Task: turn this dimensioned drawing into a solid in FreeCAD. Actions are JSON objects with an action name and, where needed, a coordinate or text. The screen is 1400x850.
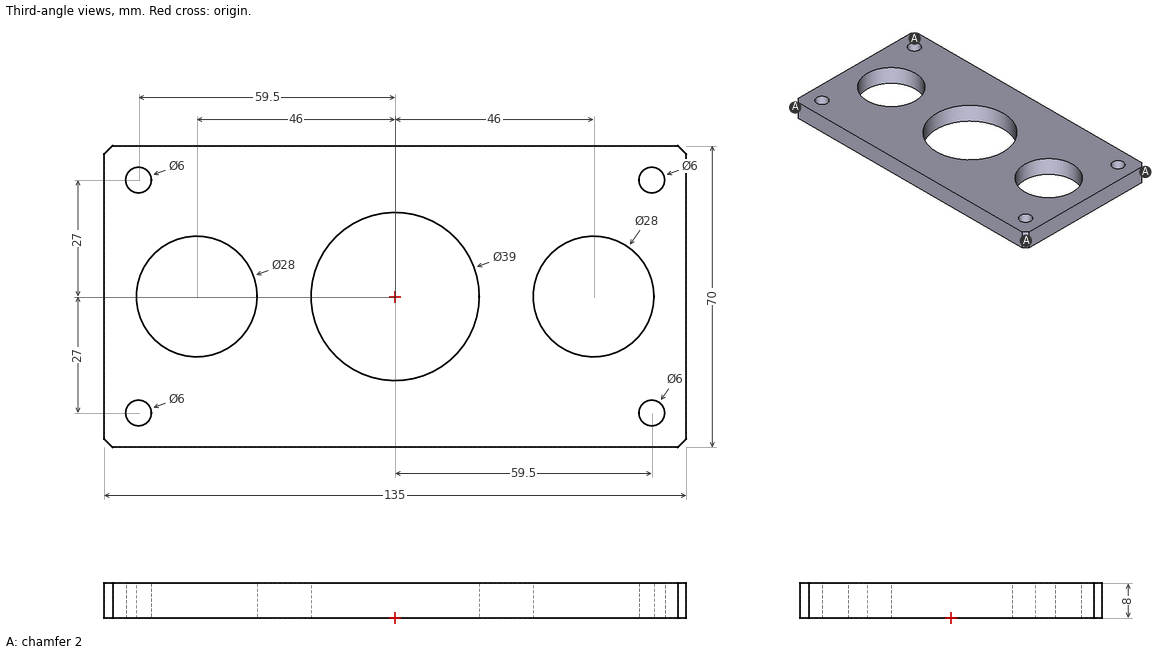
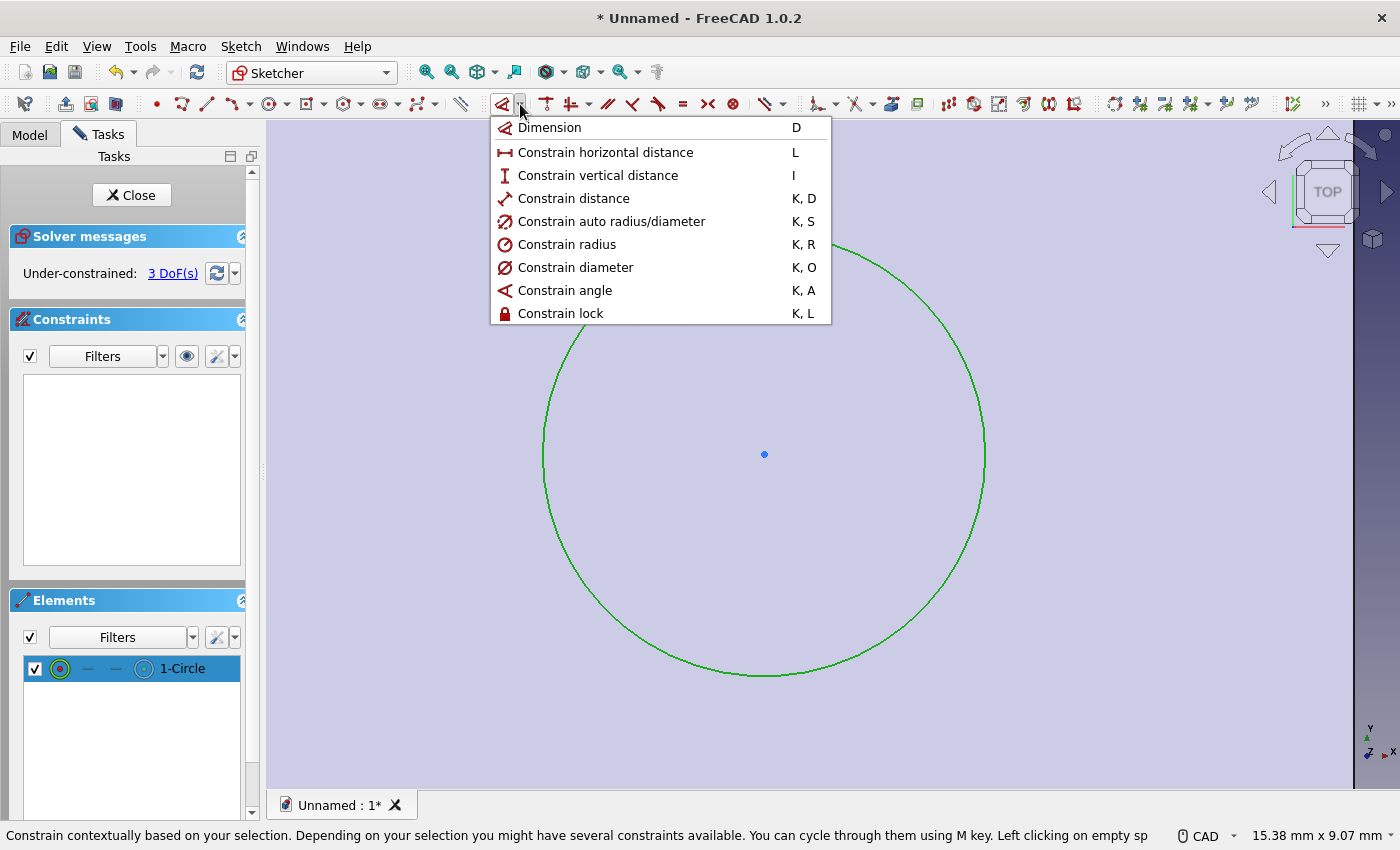
{"action": "left_click", "coordinate": [661, 268]}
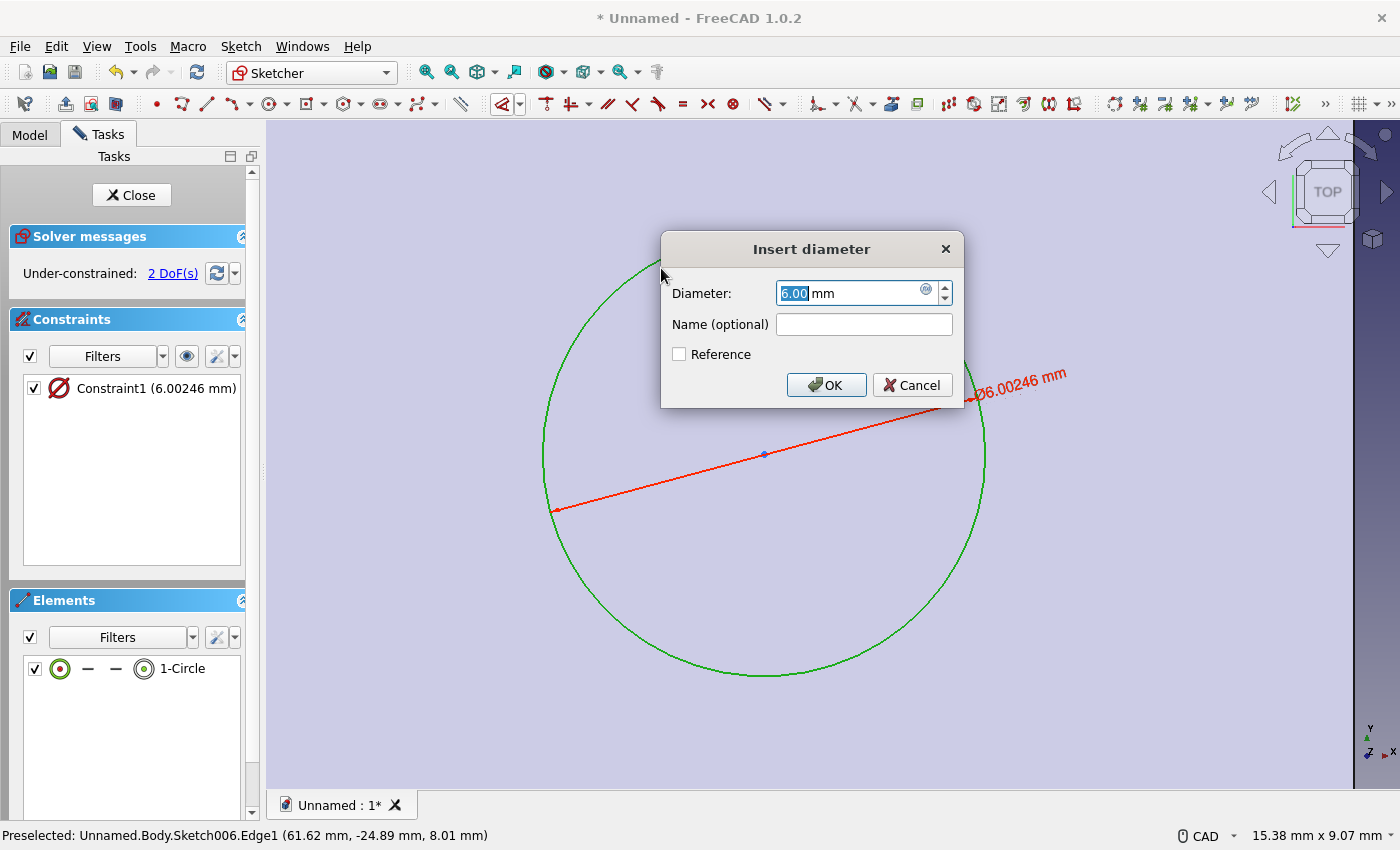
{"action": "type", "text": "6"}
{"action": "key", "text": "Return"}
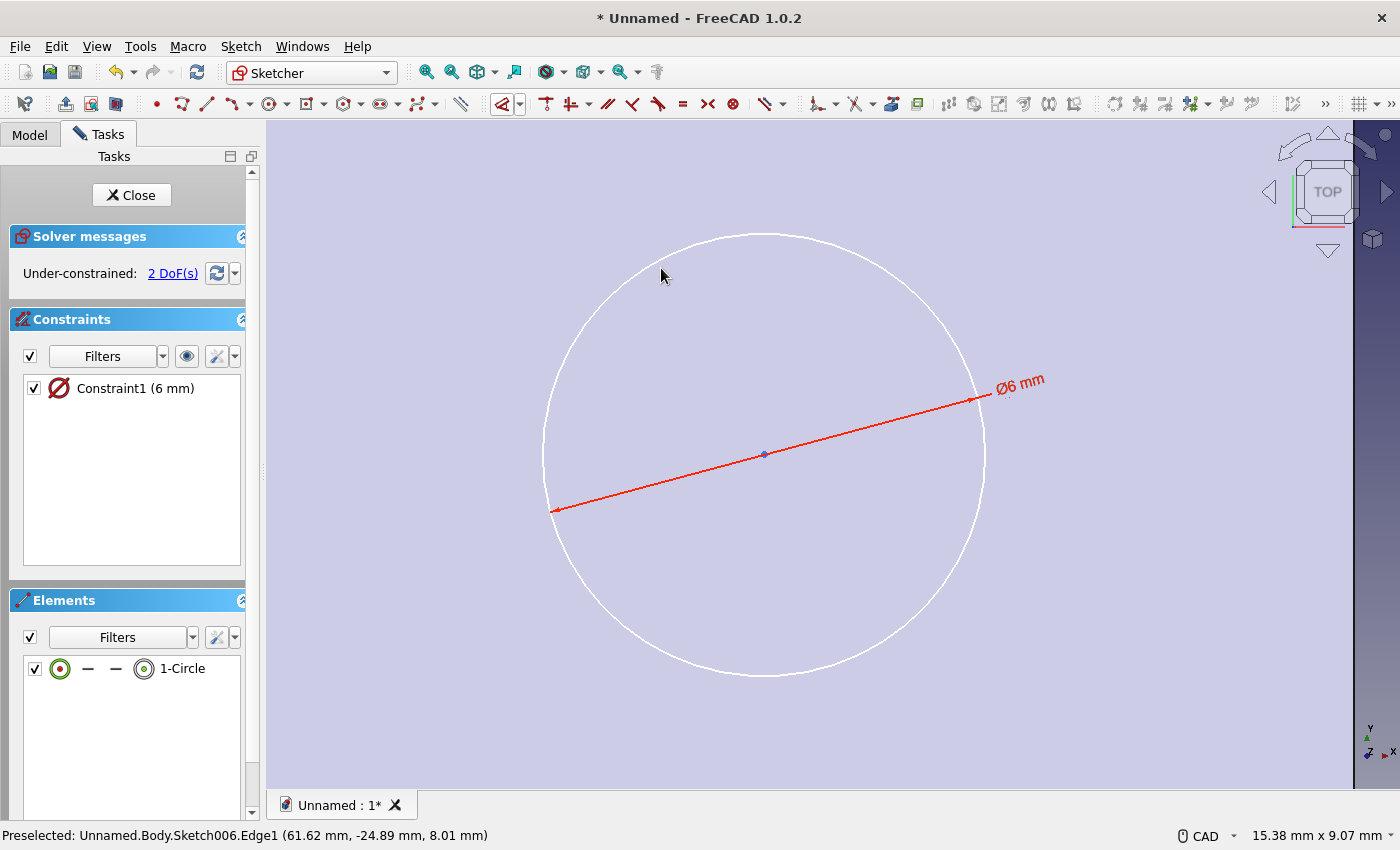
{"action": "left_click", "coordinate": [764, 455]}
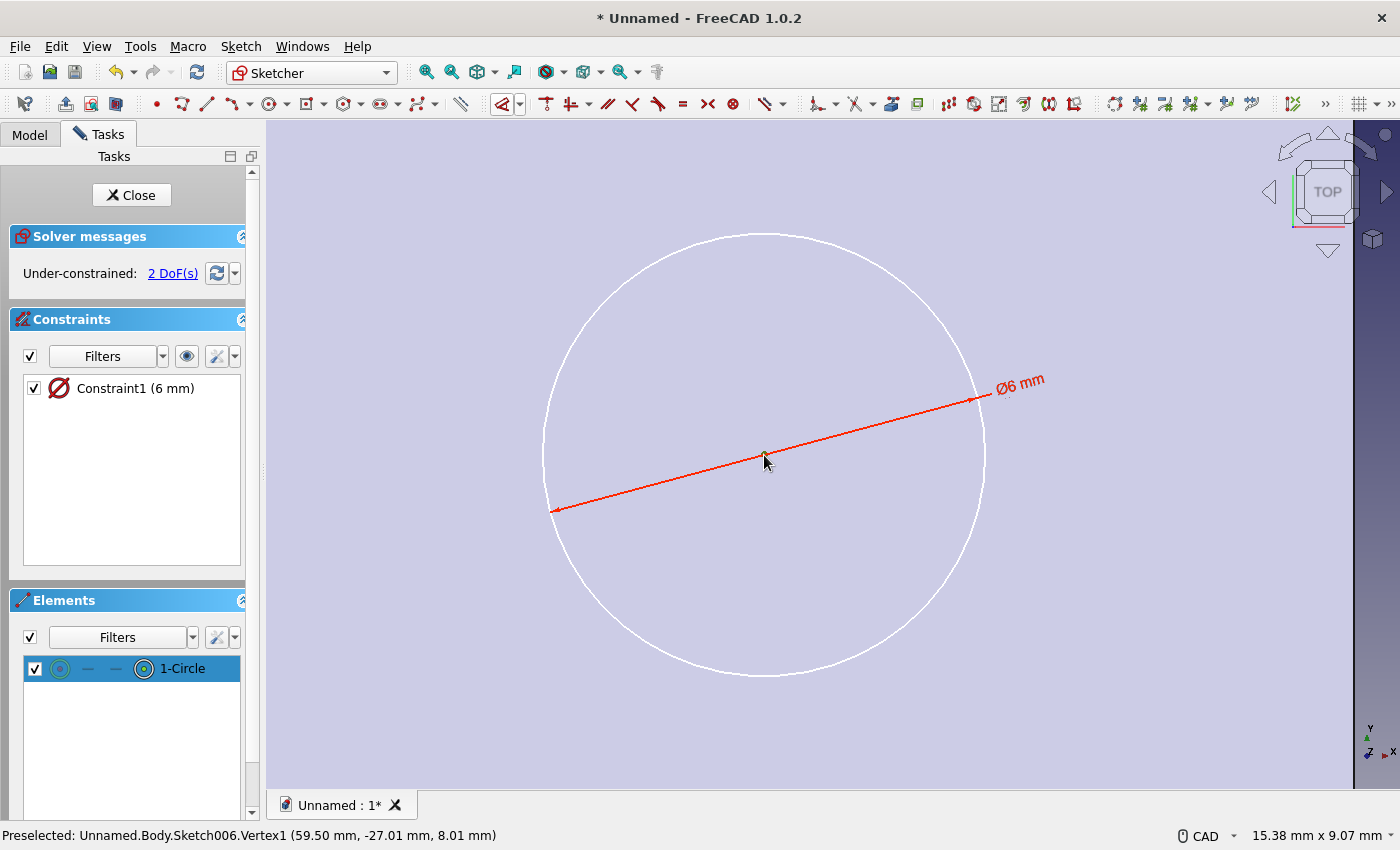
{"action": "key", "text": "i"}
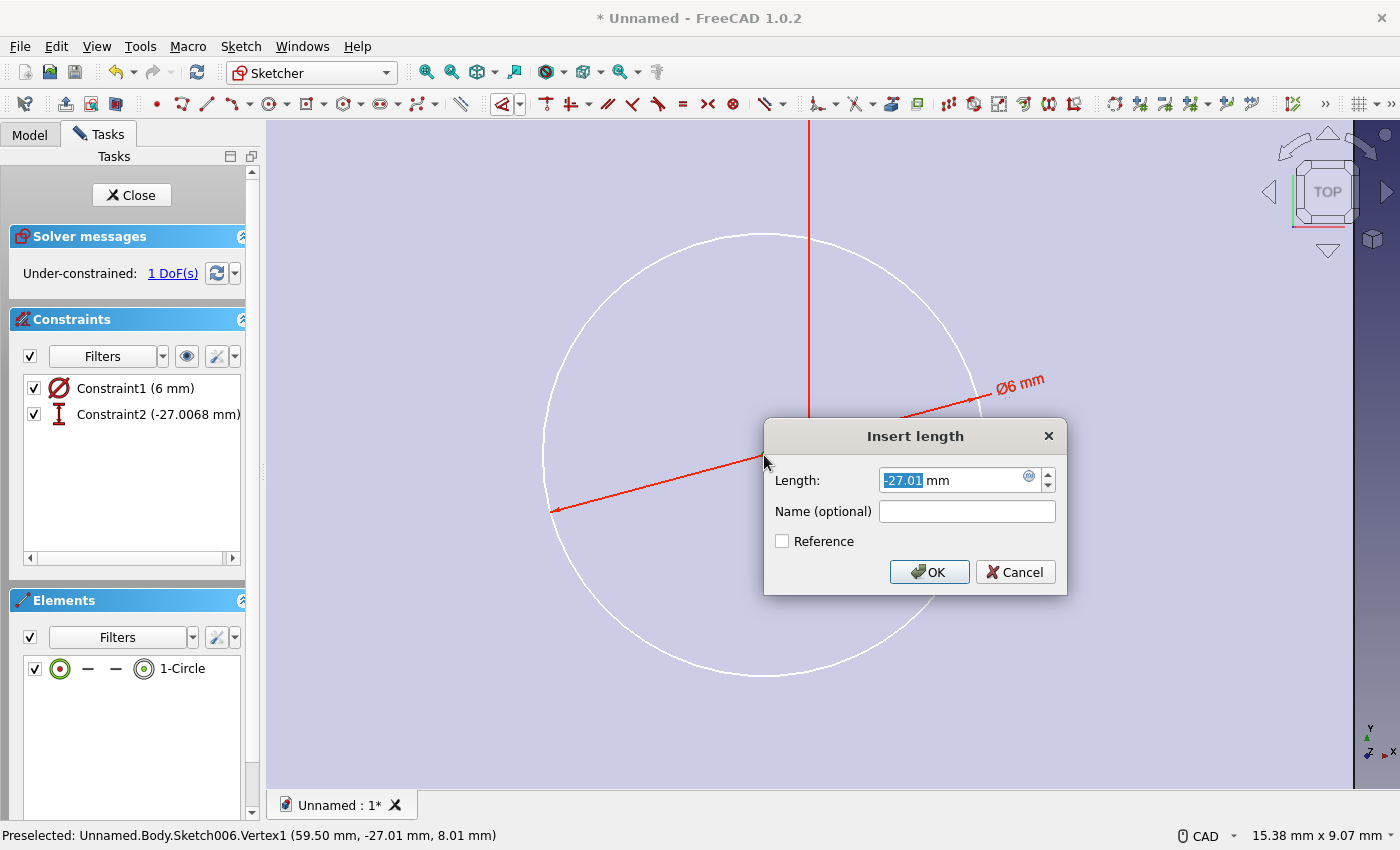
{"action": "type", "text": "-27"}
{"action": "key", "text": "Return"}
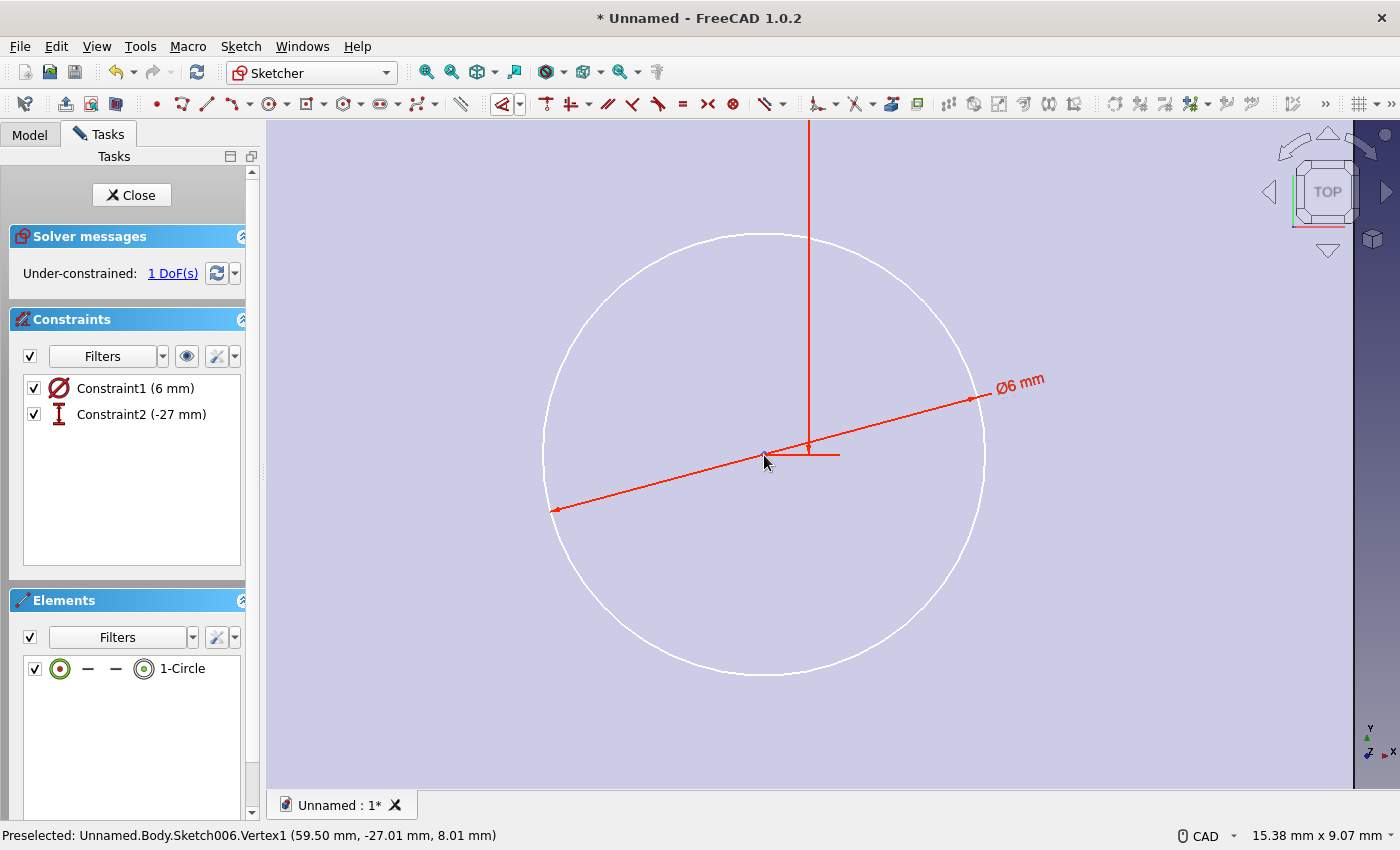
{"action": "left_click", "coordinate": [764, 454]}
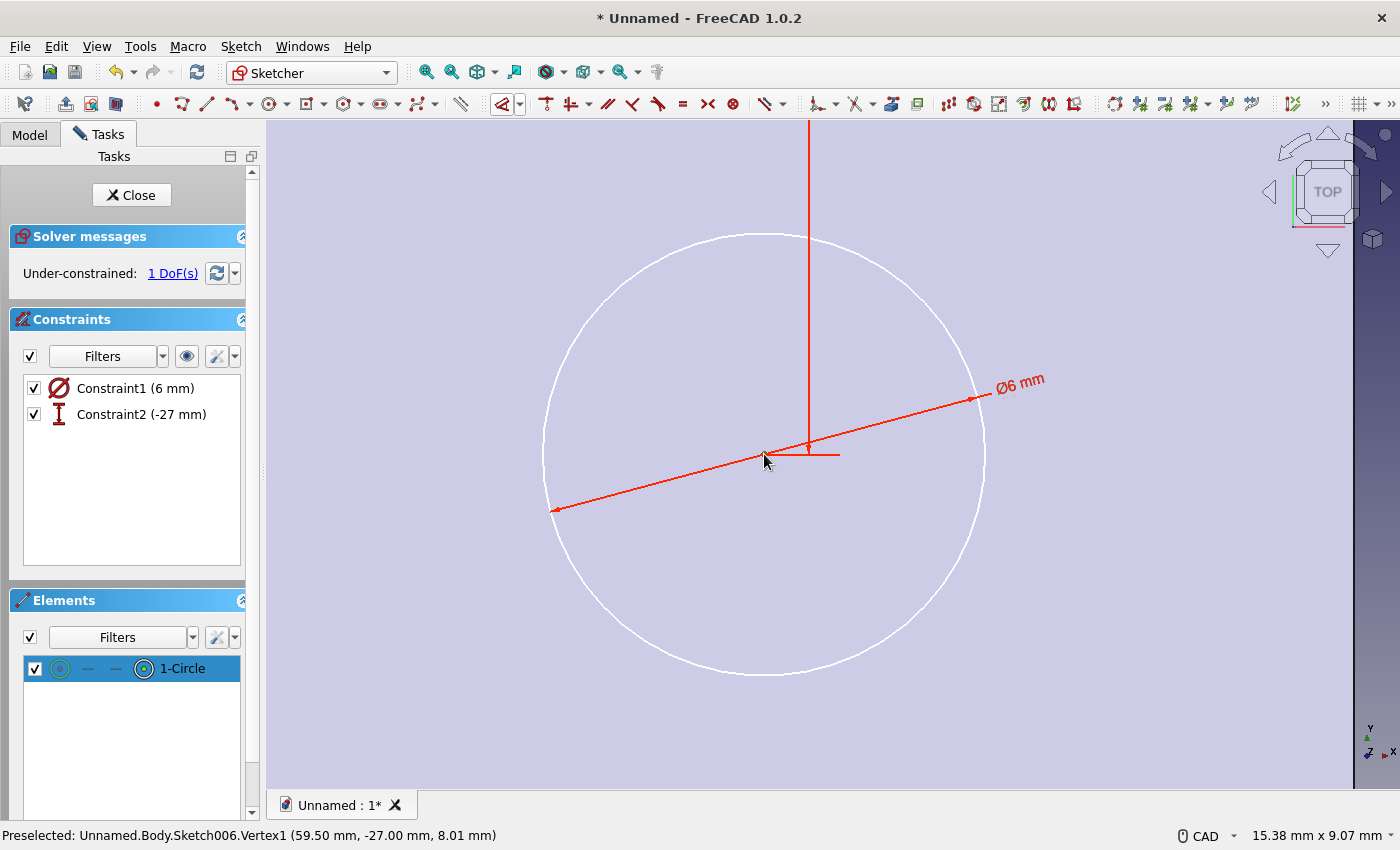
{"action": "key", "text": "l"}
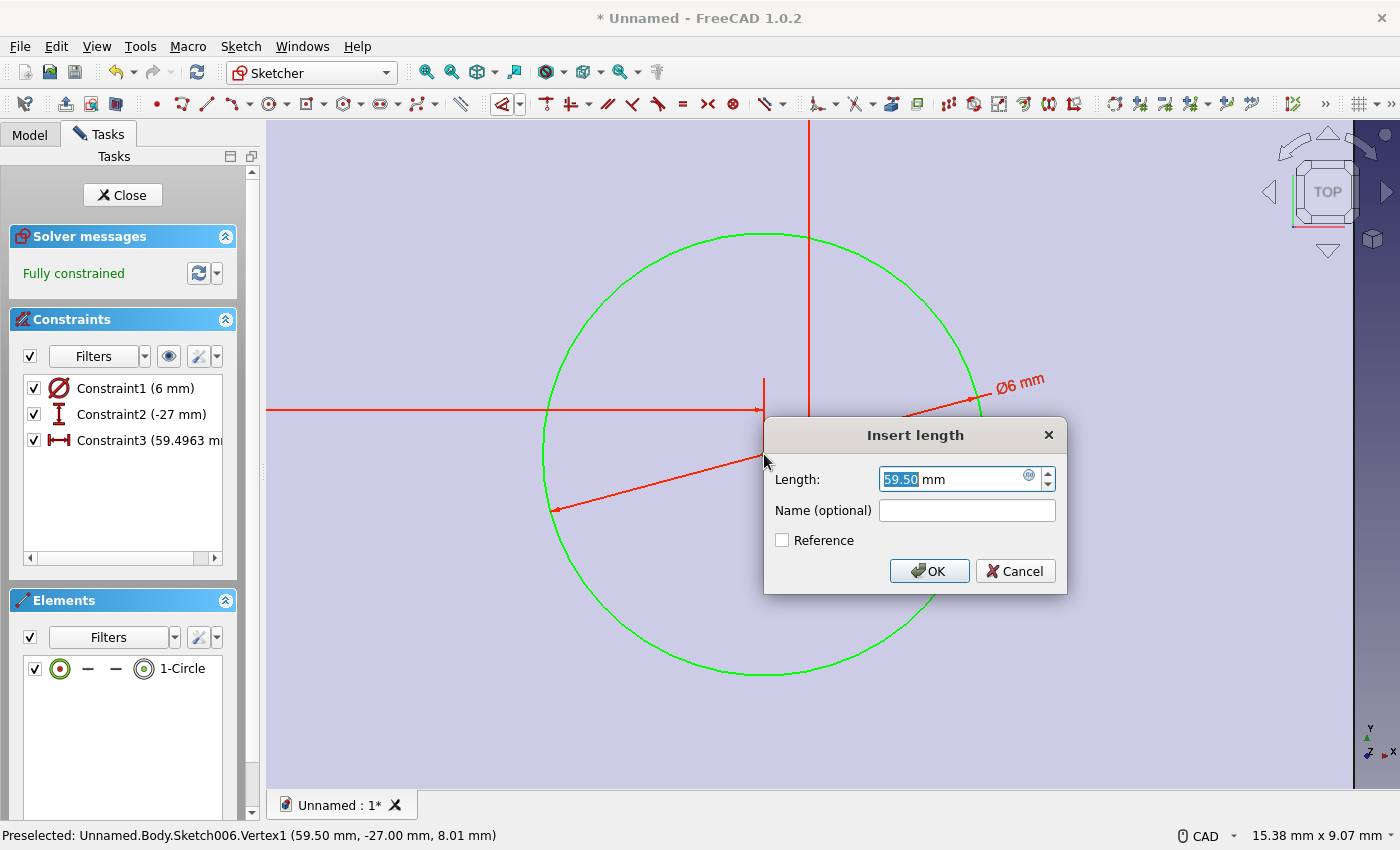
{"action": "type", "text": "59.5"}
{"action": "key", "text": "Return"}